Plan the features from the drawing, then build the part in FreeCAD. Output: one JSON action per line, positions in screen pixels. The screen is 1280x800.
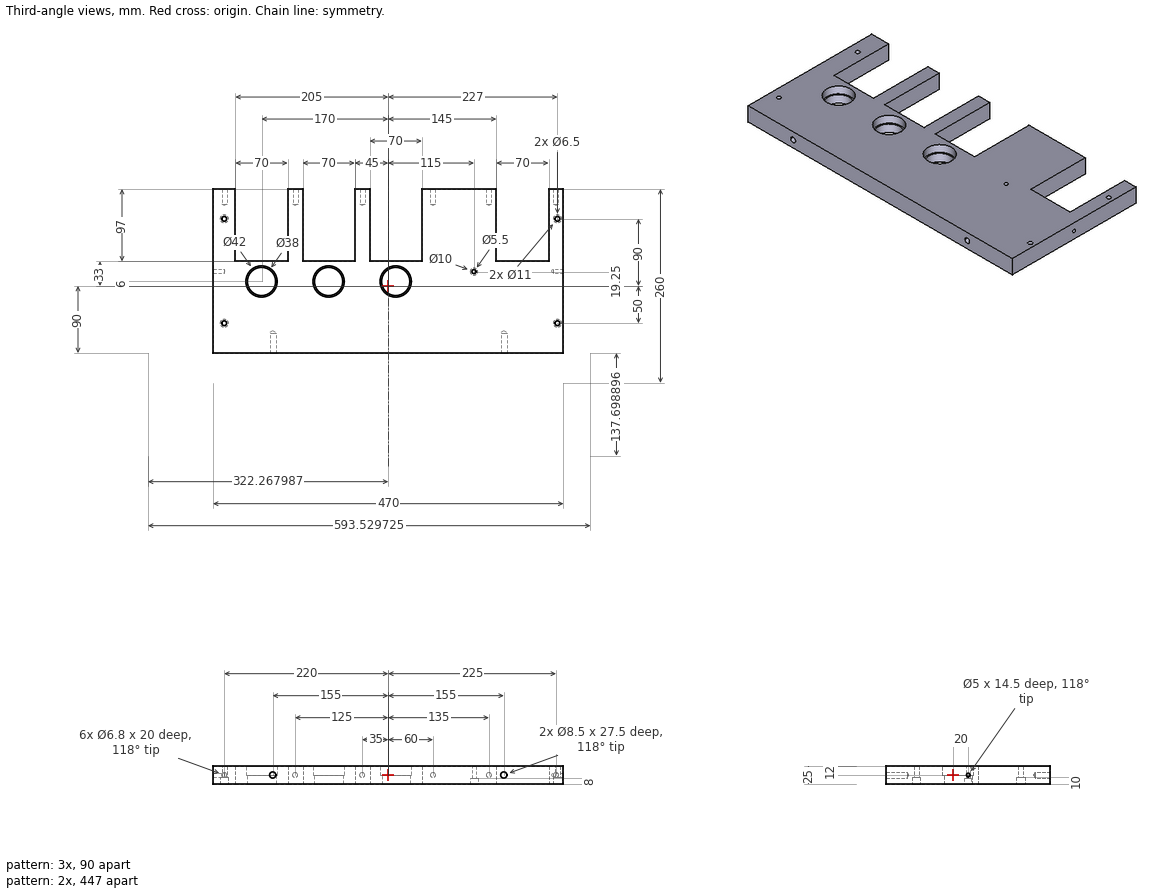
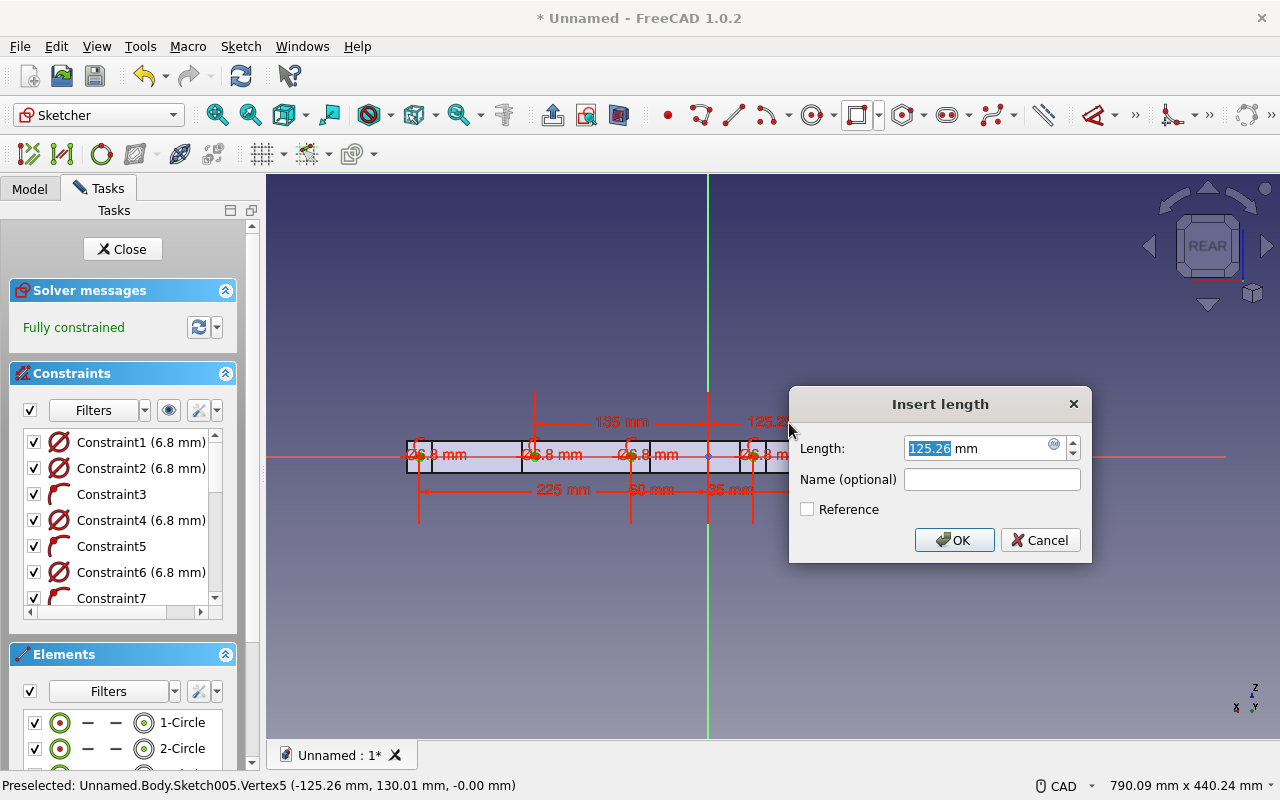
{"action": "type", "text": "125"}
{"action": "key", "text": "Return"}
{"action": "key", "text": "Escape"}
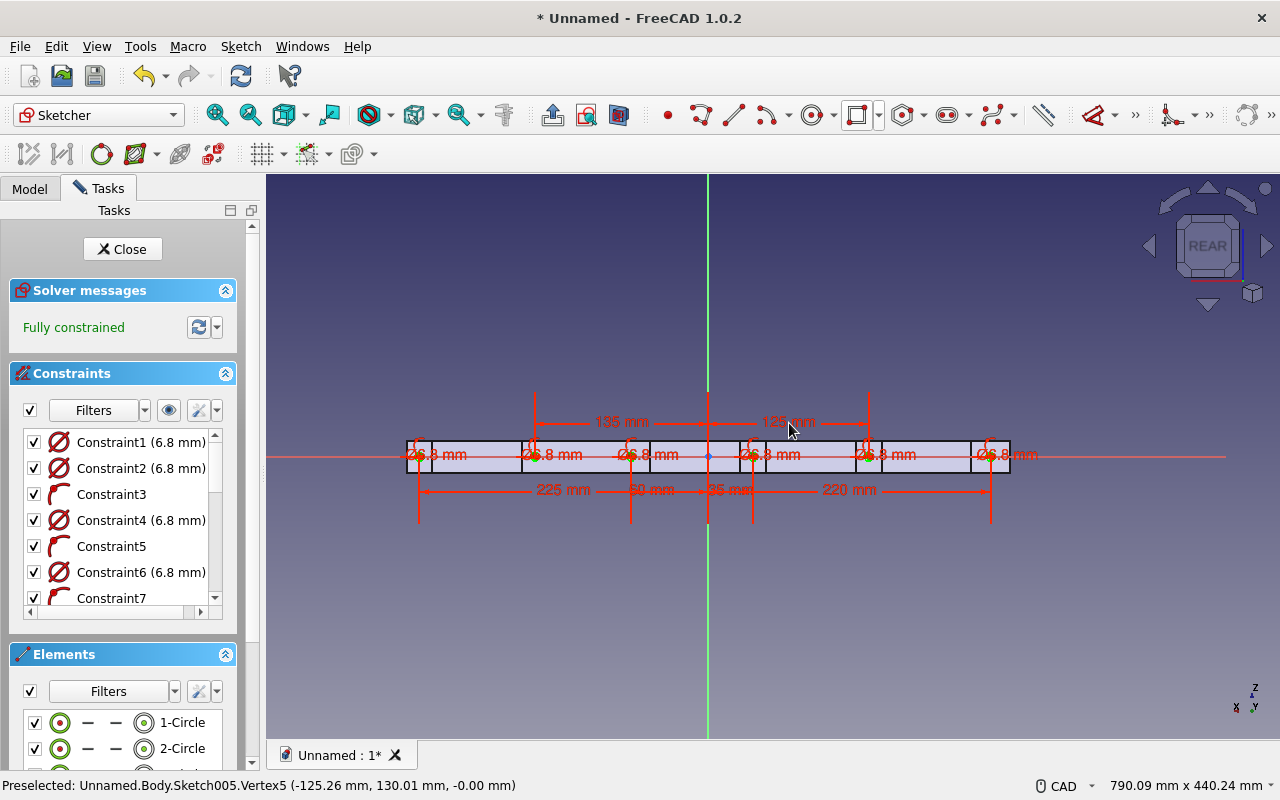
{"action": "left_click", "coordinate": [123, 249]}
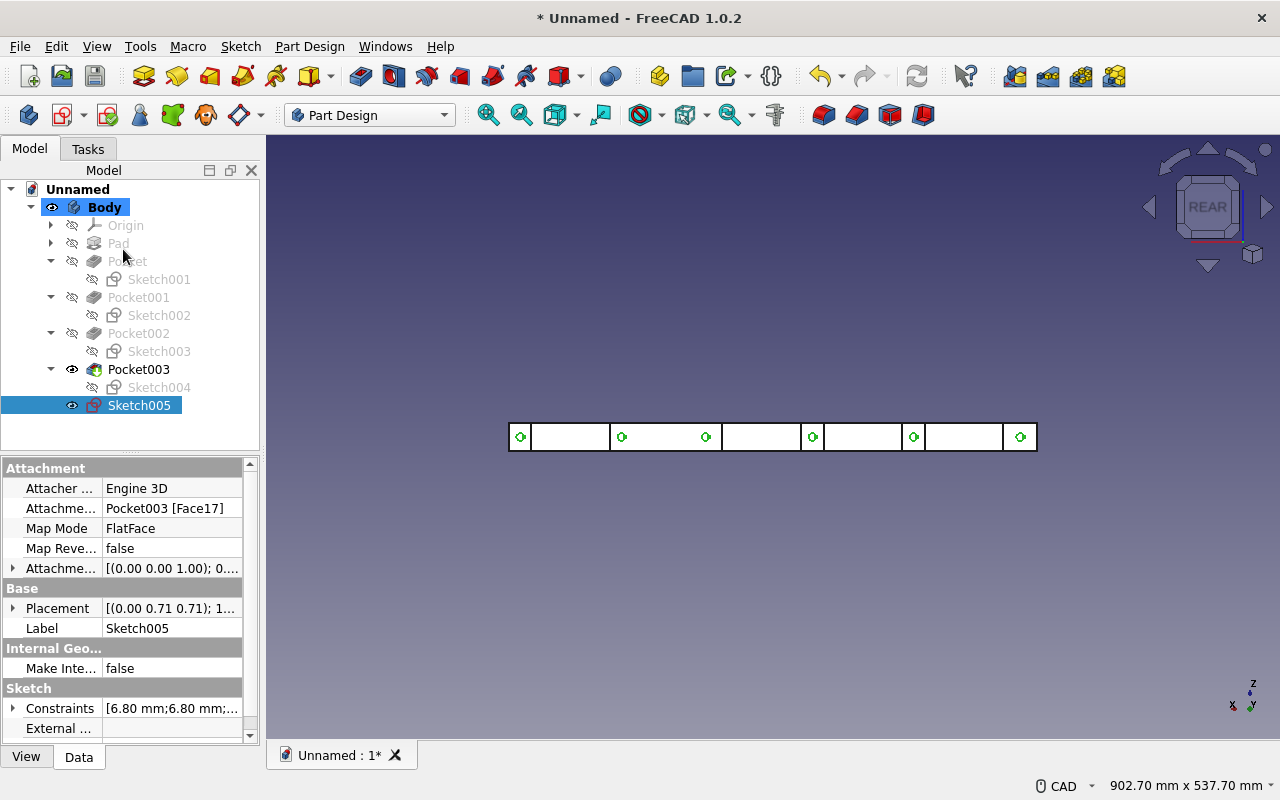
{"action": "left_click", "coordinate": [394, 76]}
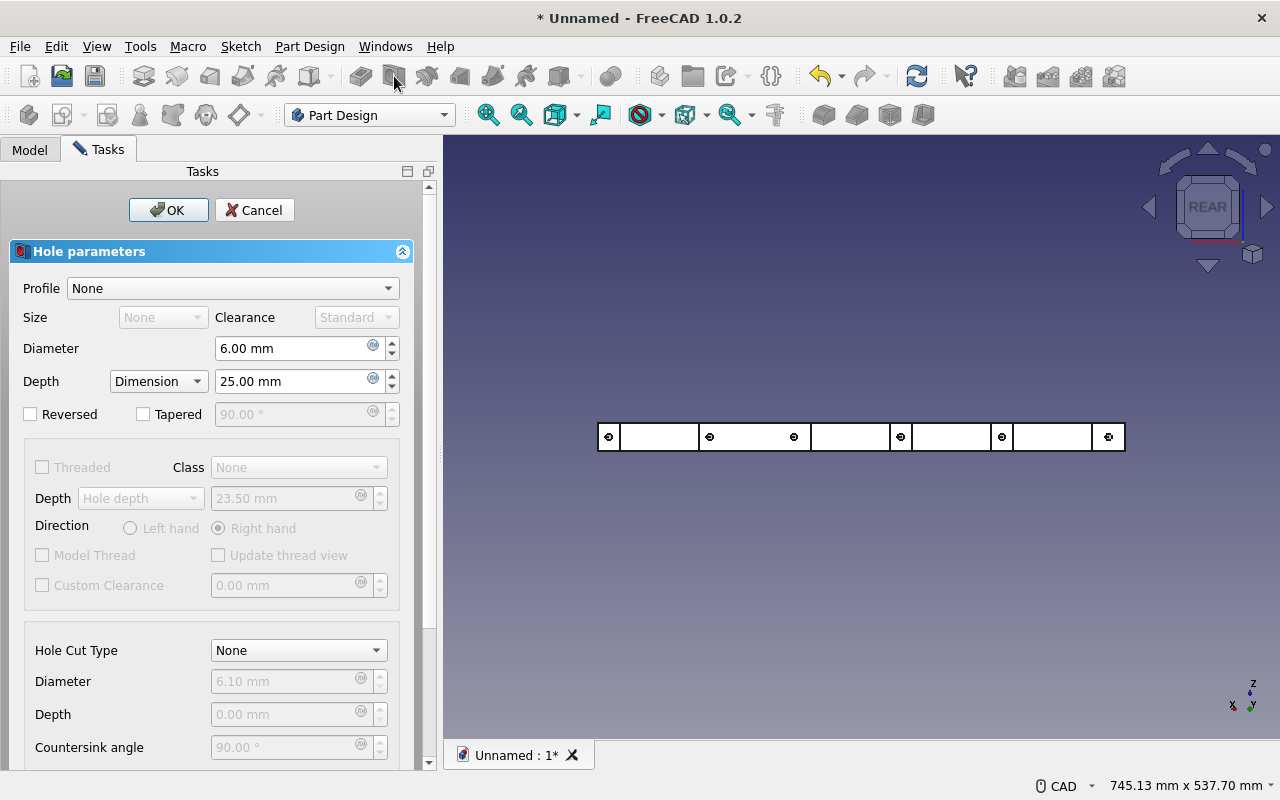
{"action": "triple_click", "coordinate": [300, 348]}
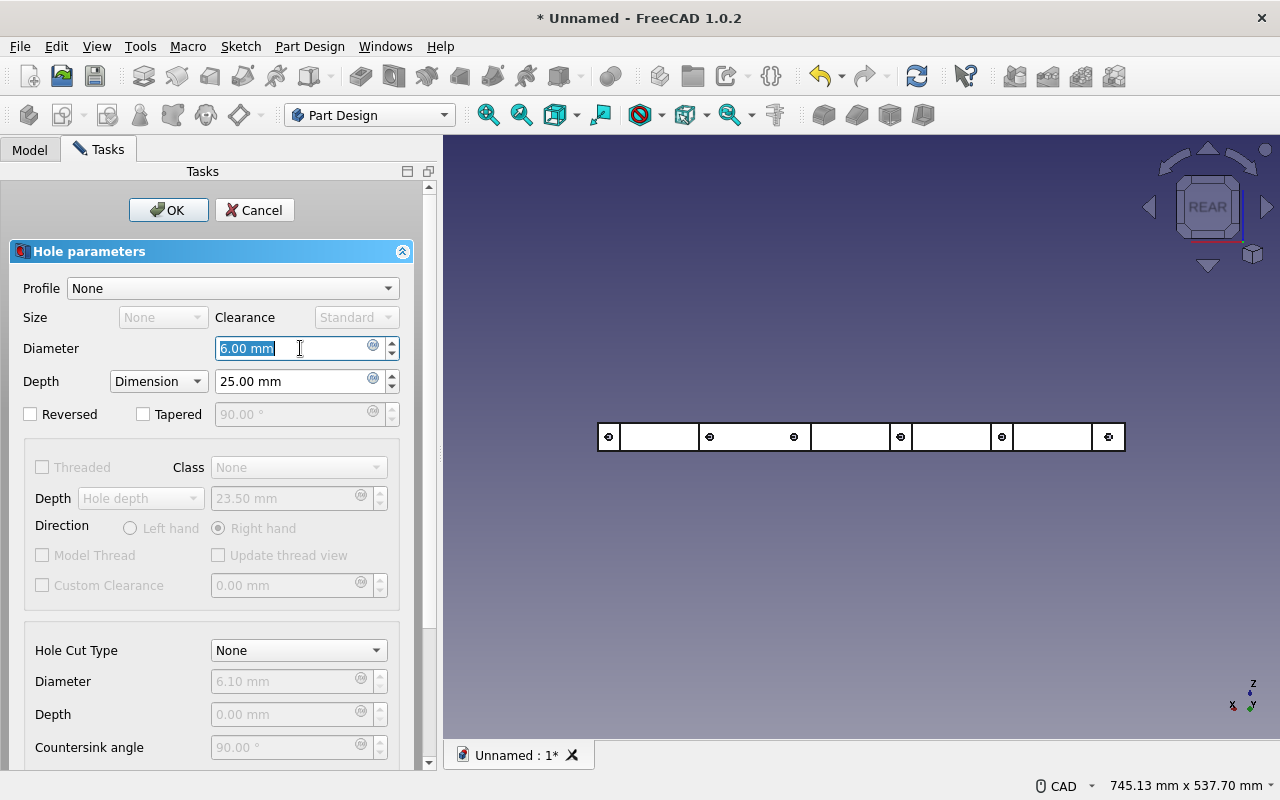
{"action": "type", "text": "6.8"}
{"action": "key", "text": "Tab"}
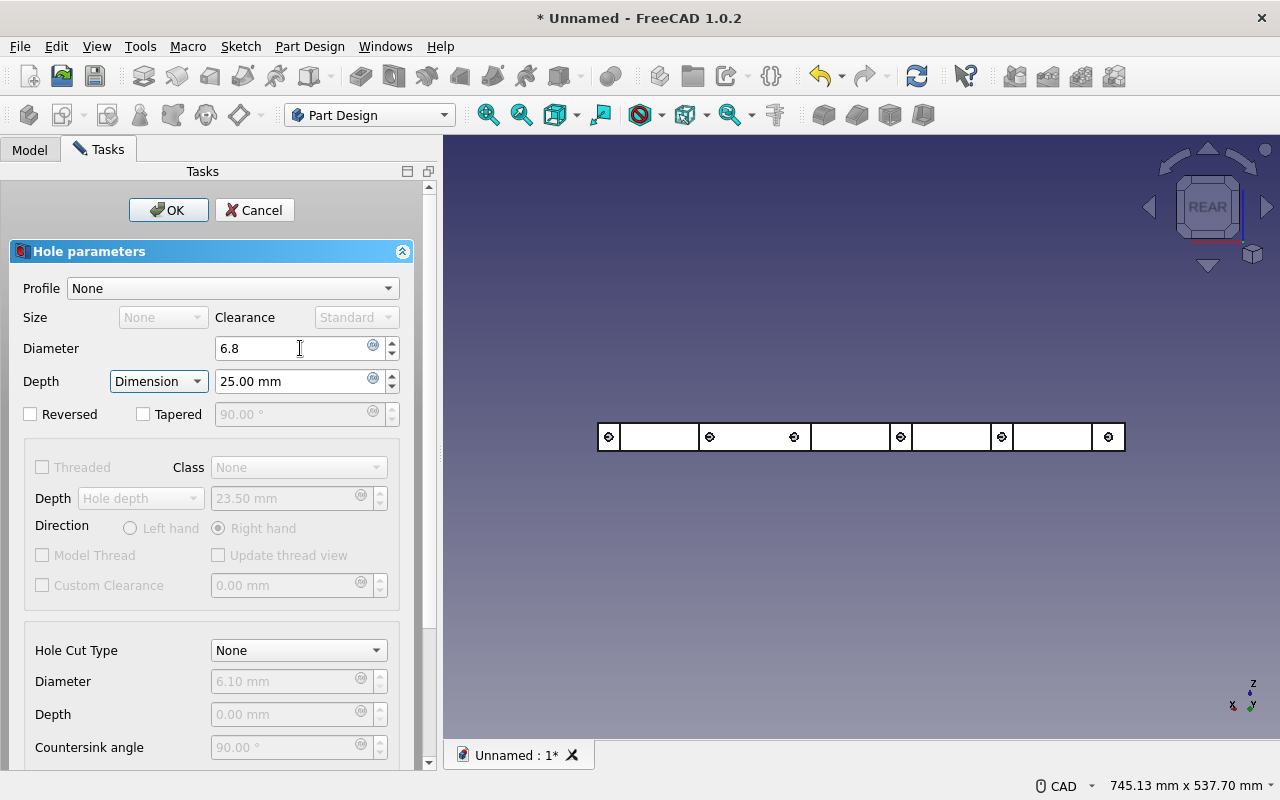
{"action": "triple_click", "coordinate": [300, 382]}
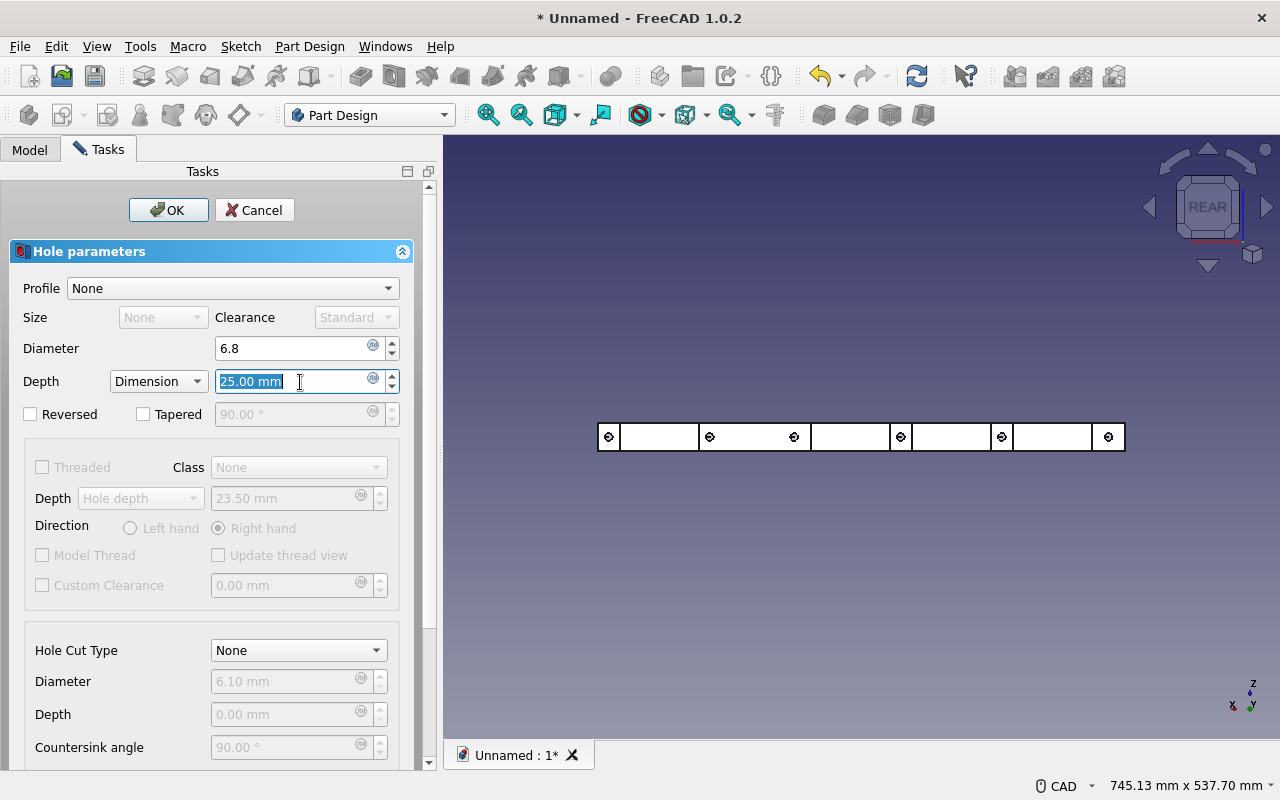
{"action": "type", "text": "20"}
{"action": "key", "text": "Tab"}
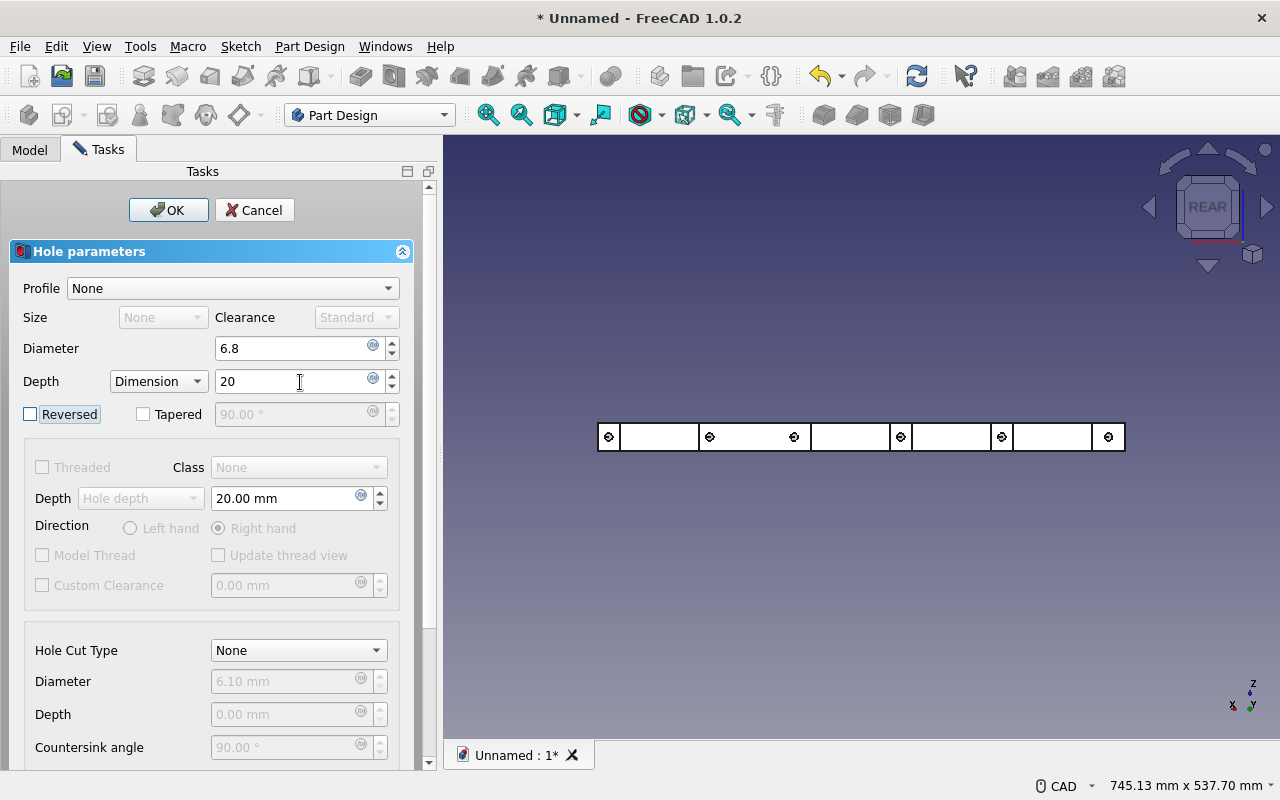
{"action": "left_click", "coordinate": [169, 210]}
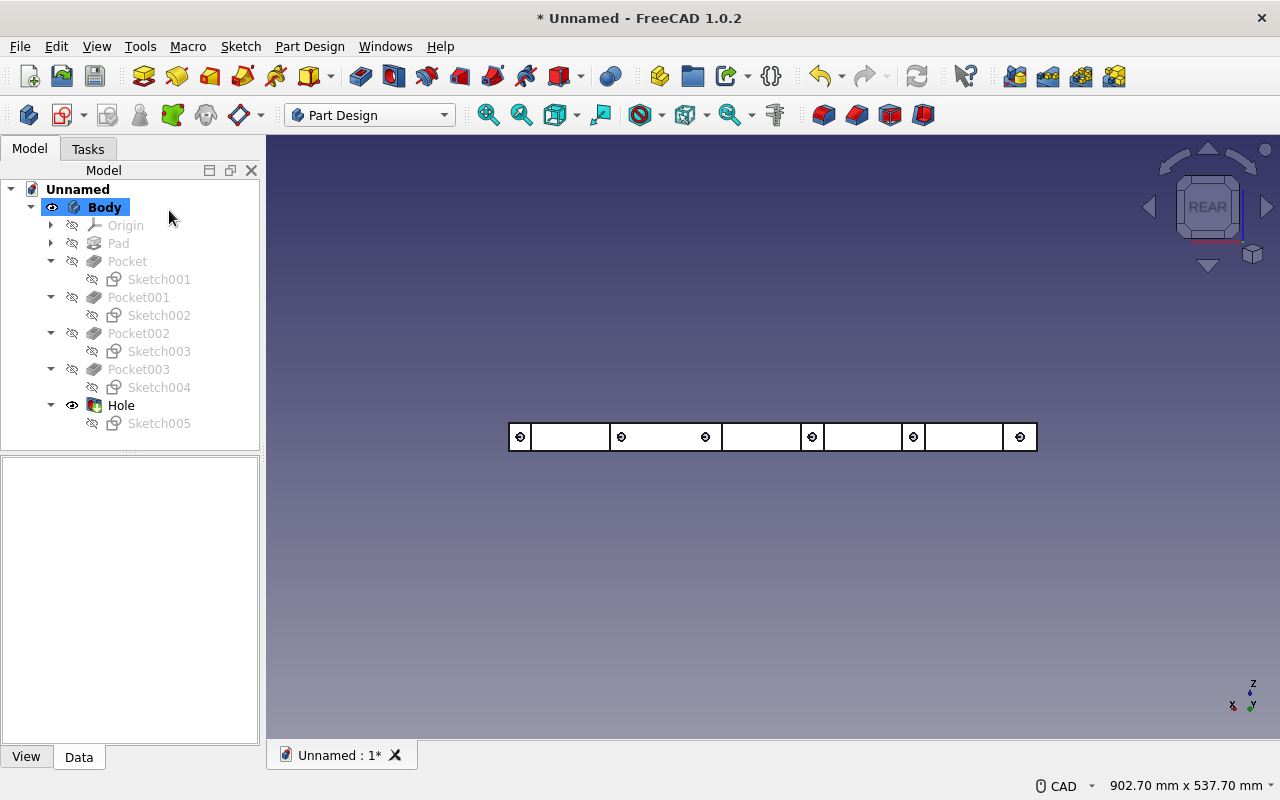
{"action": "key", "text": "0"}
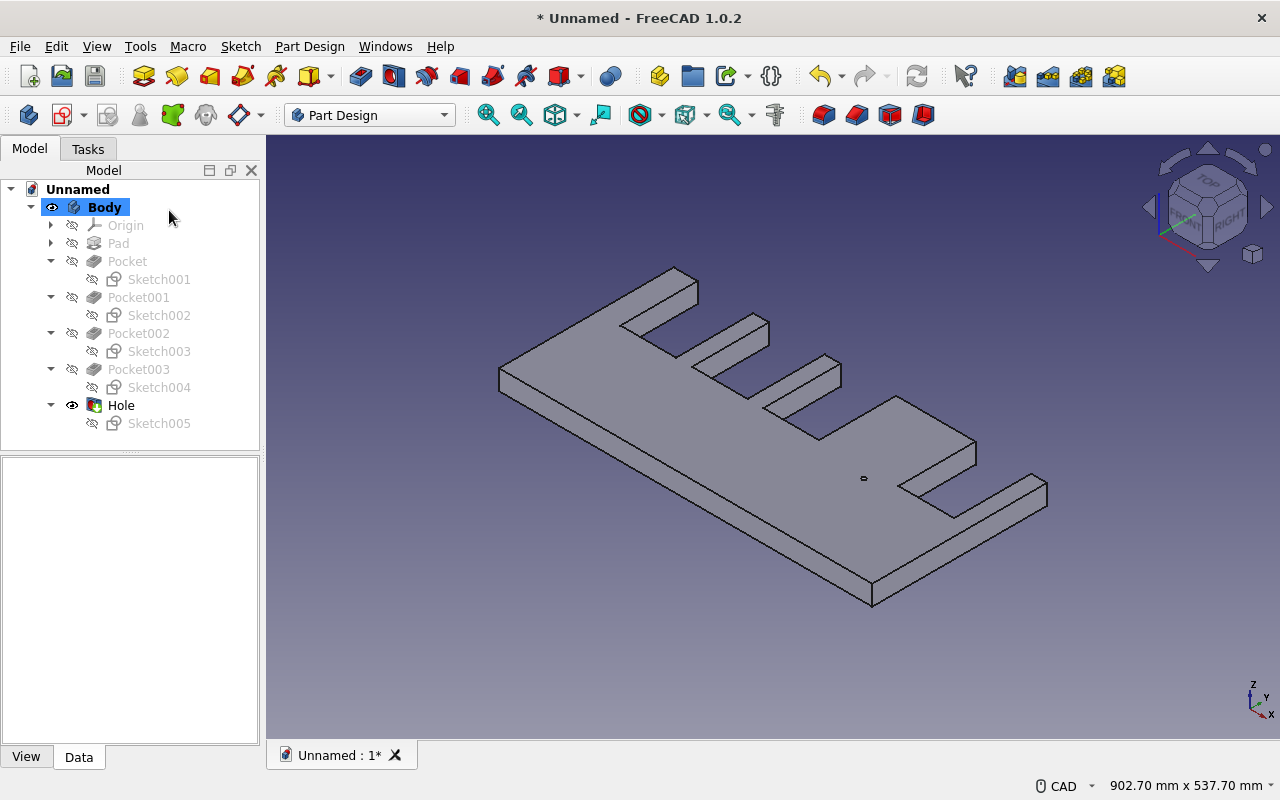
{"action": "left_click", "coordinate": [846, 579]}